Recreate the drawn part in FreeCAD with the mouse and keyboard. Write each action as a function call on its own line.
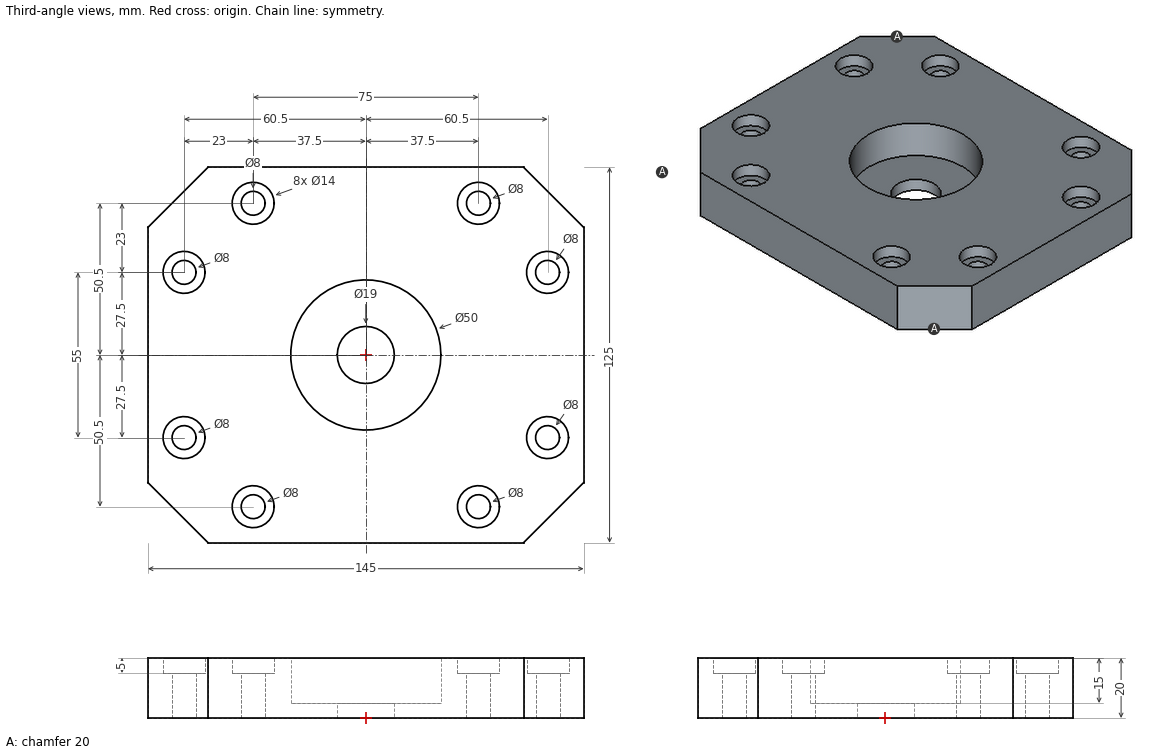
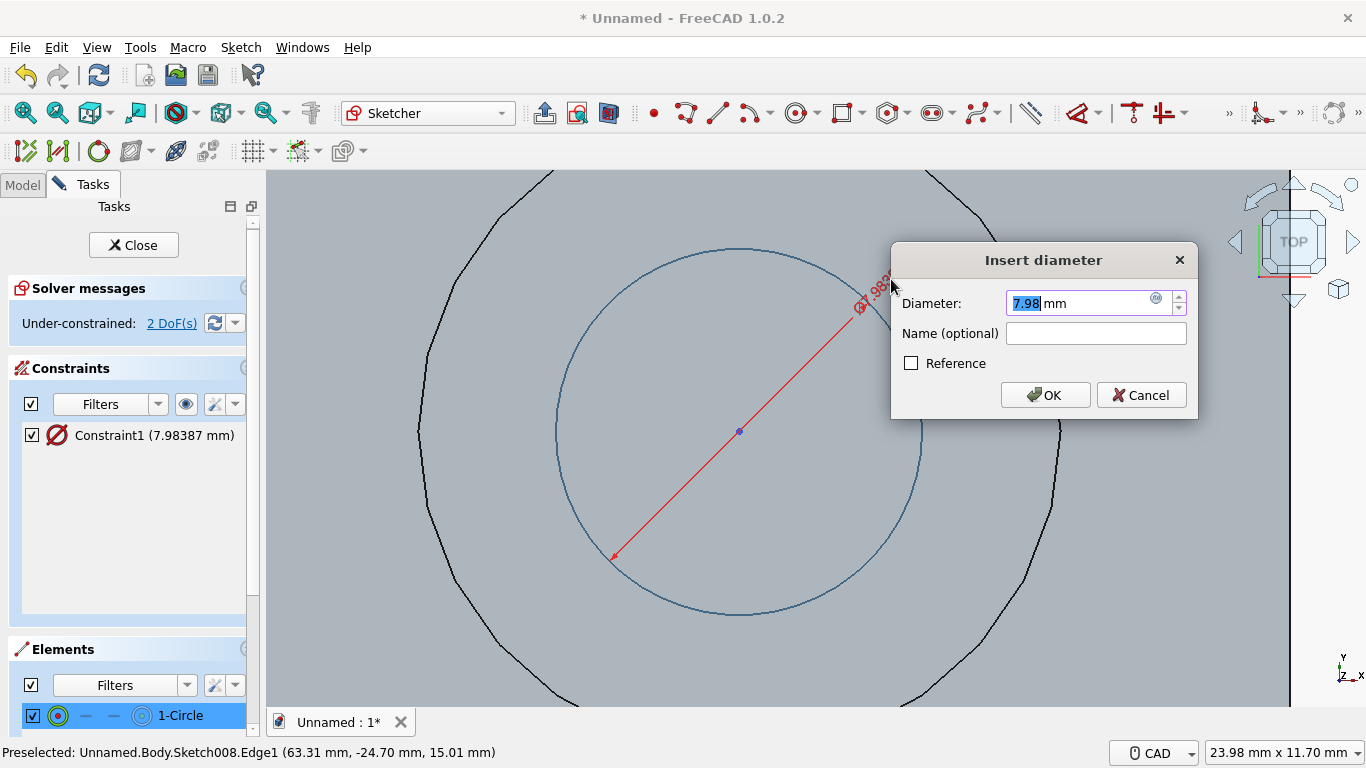
text(8)
key(Return)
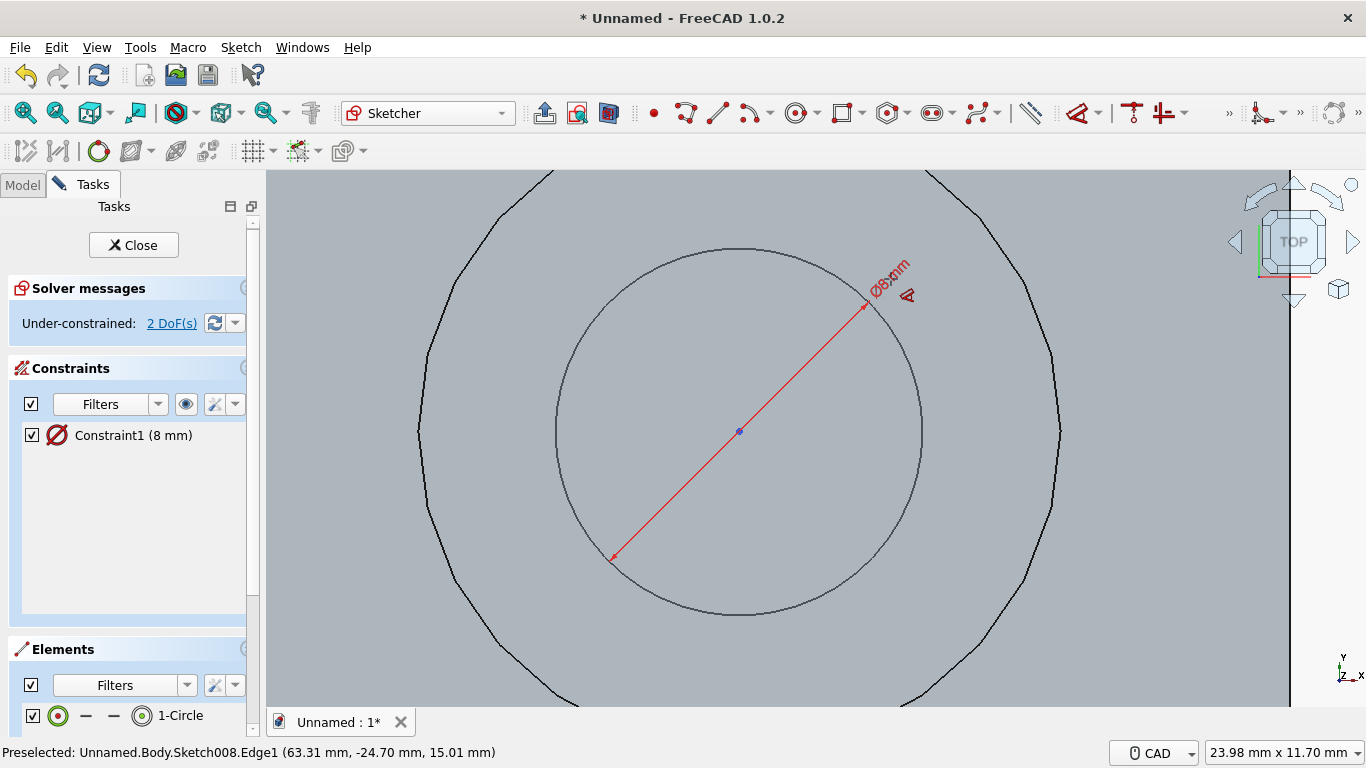
click(739, 432)
click(516, 466)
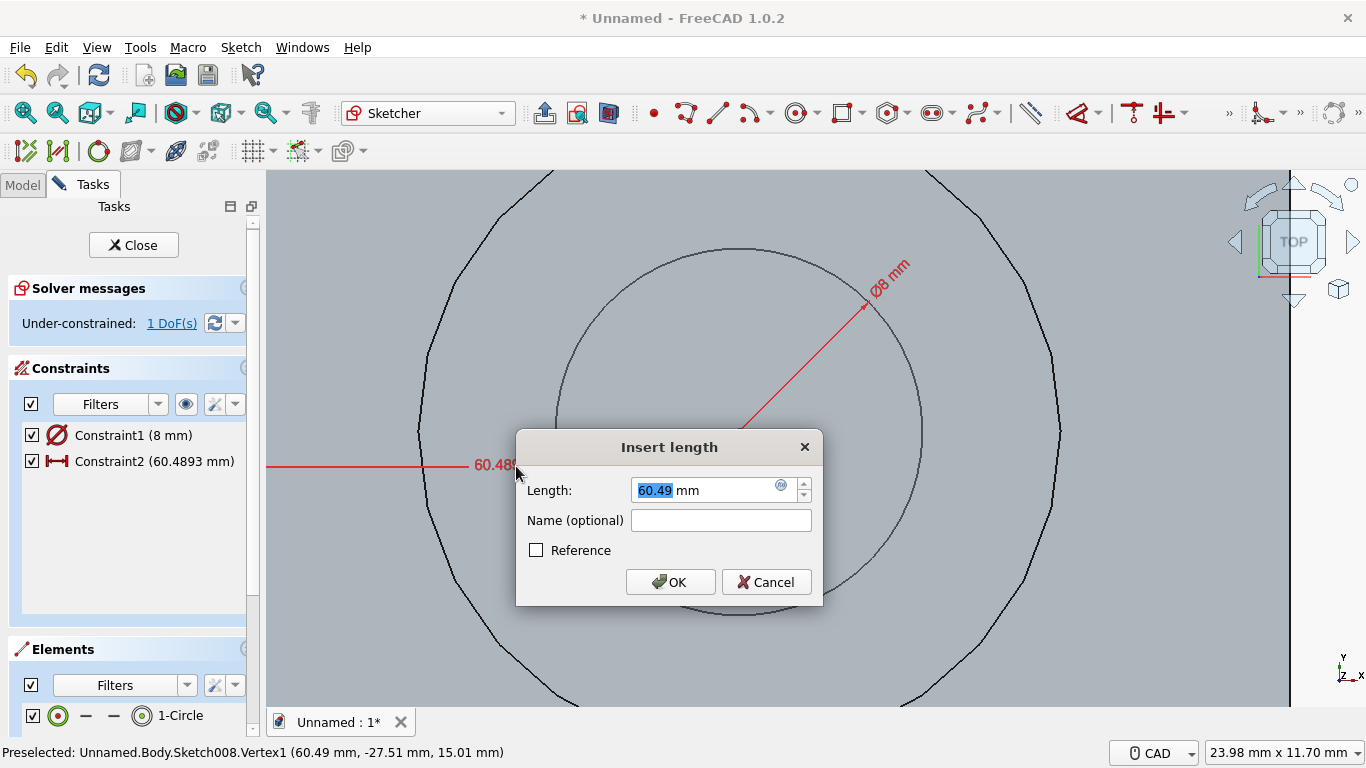
text(60.5)
key(Return)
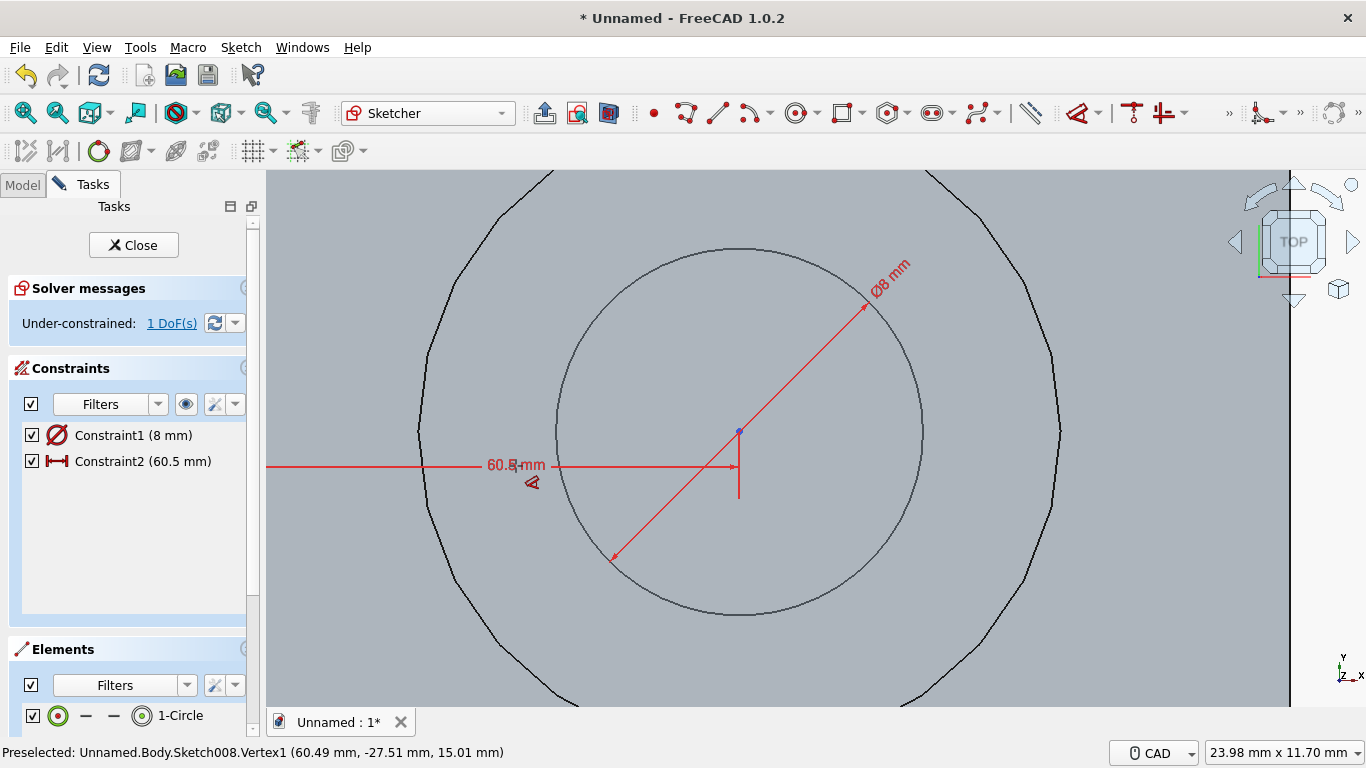
click(739, 432)
click(773, 315)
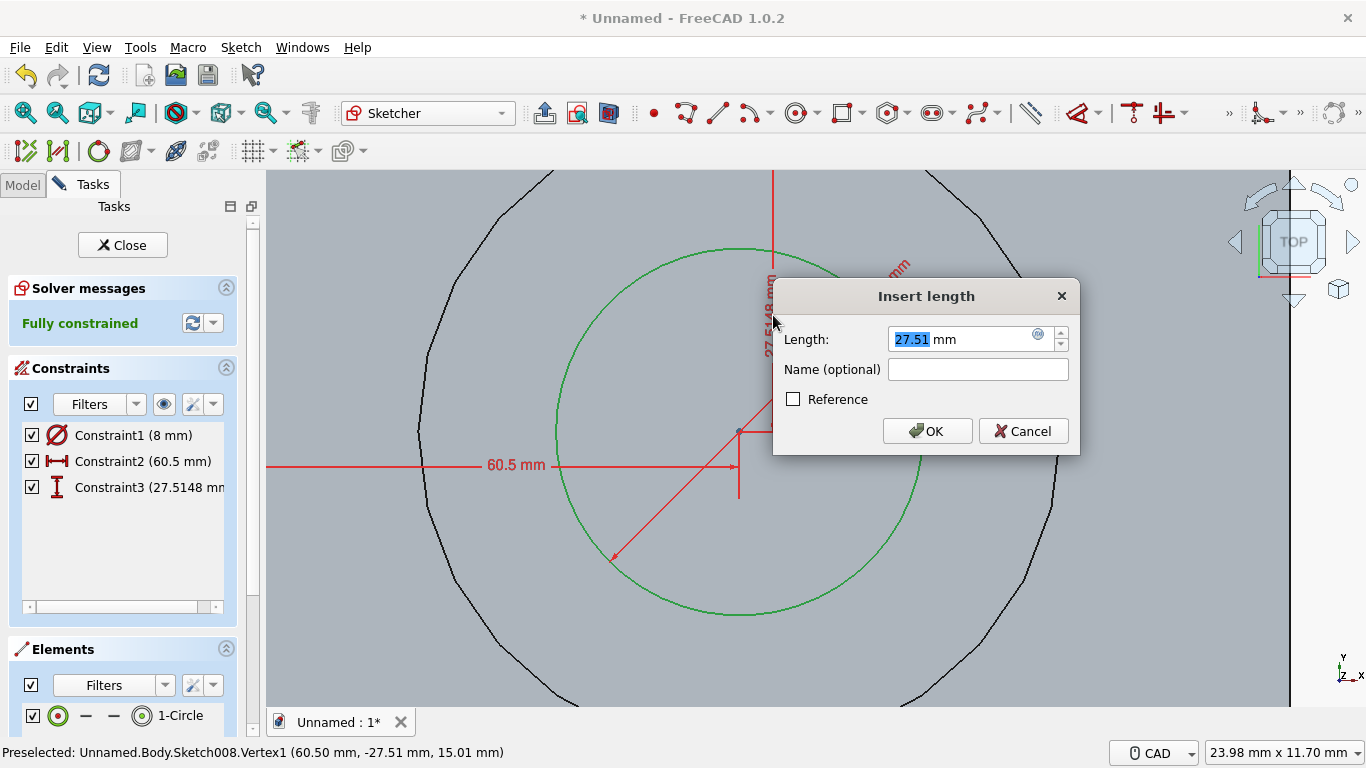
text(27.5)
key(Return)
key(Escape)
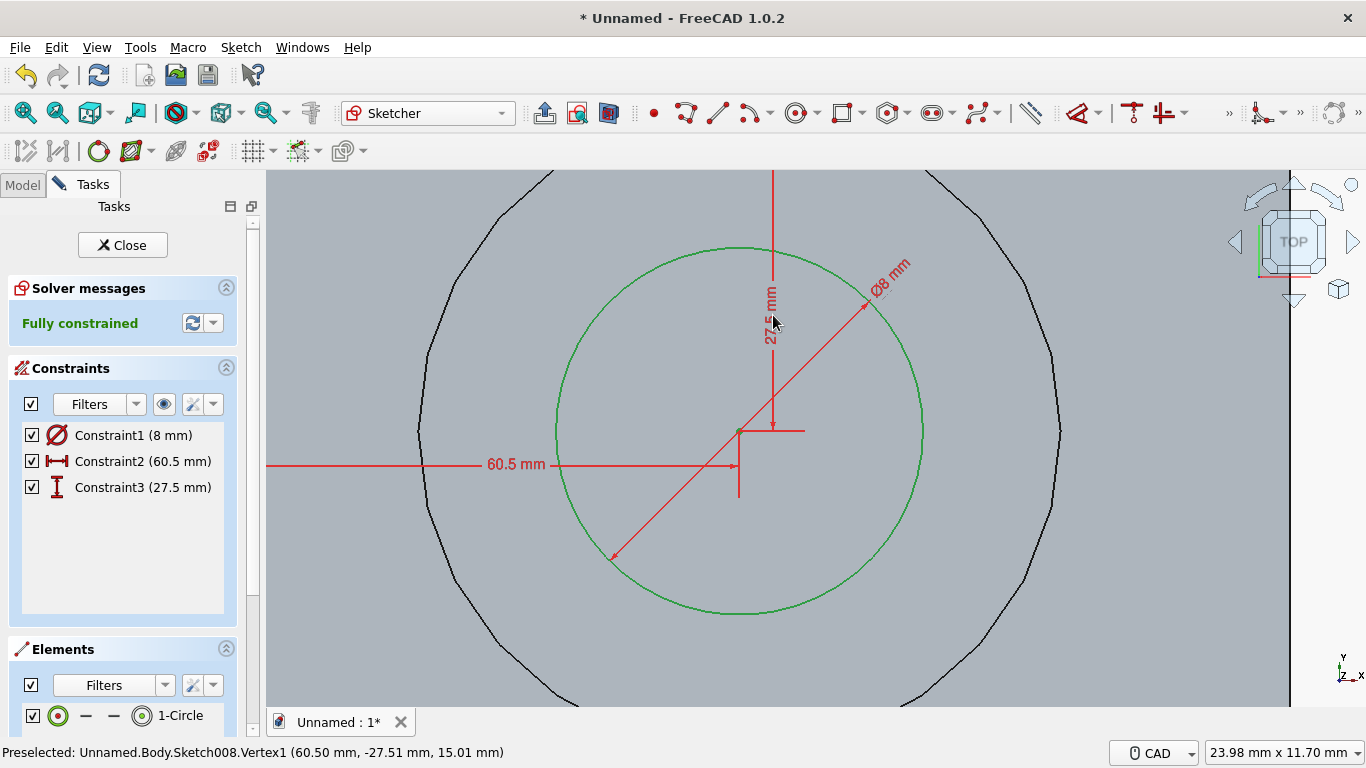
click(123, 245)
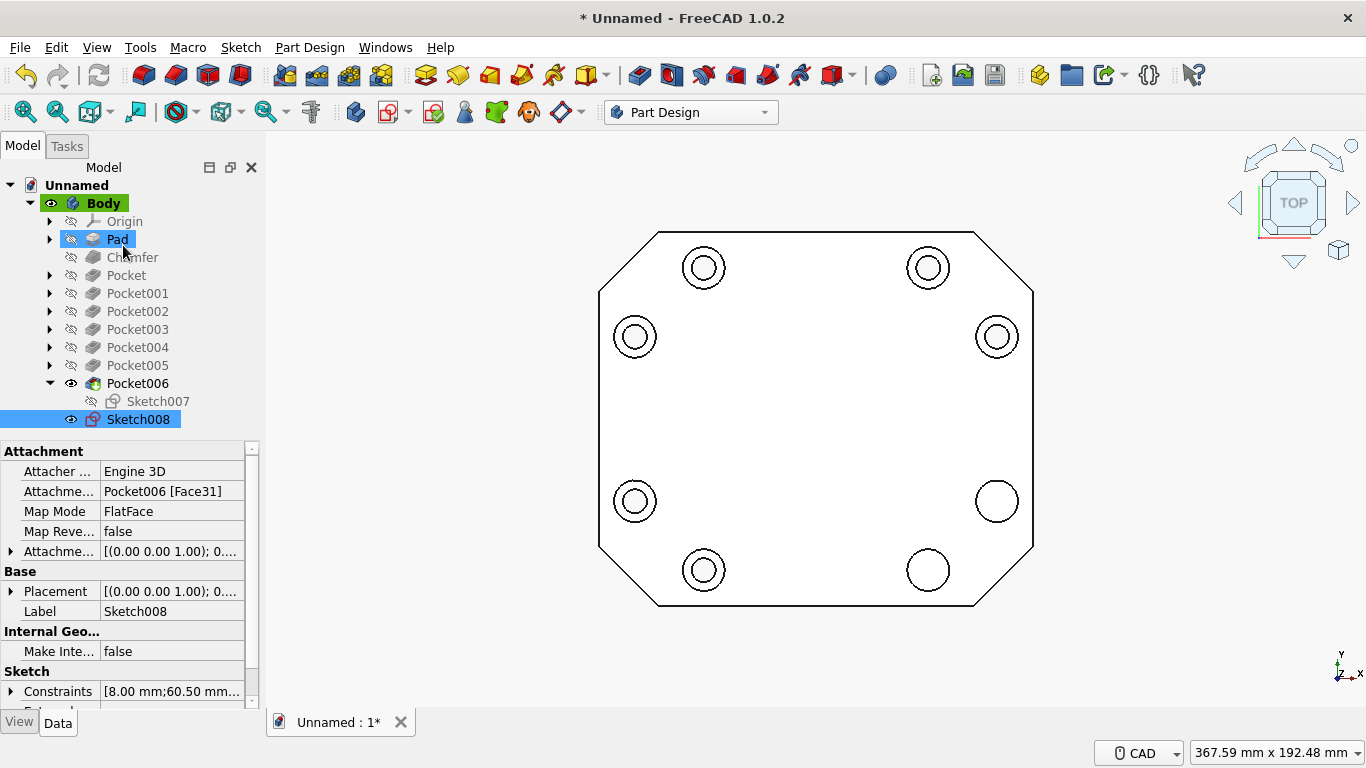
click(640, 76)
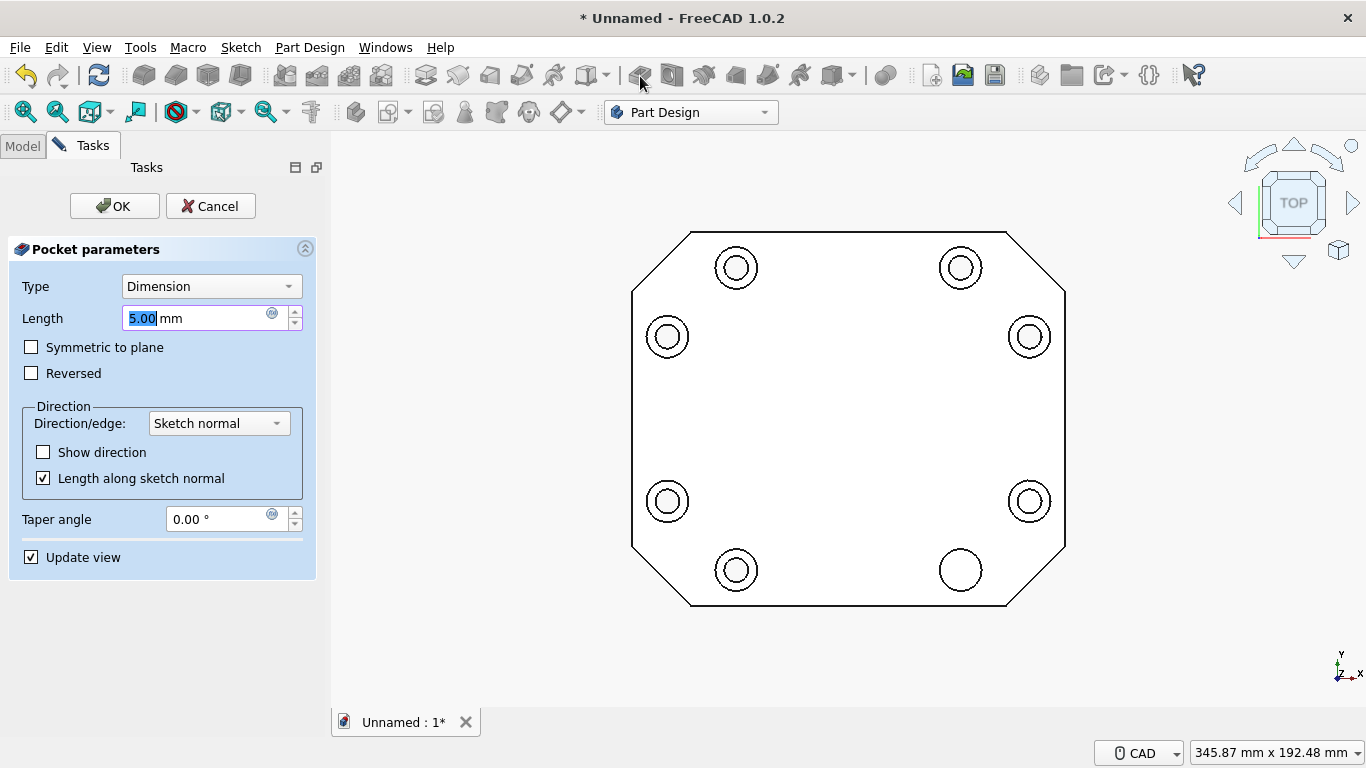
click(212, 286)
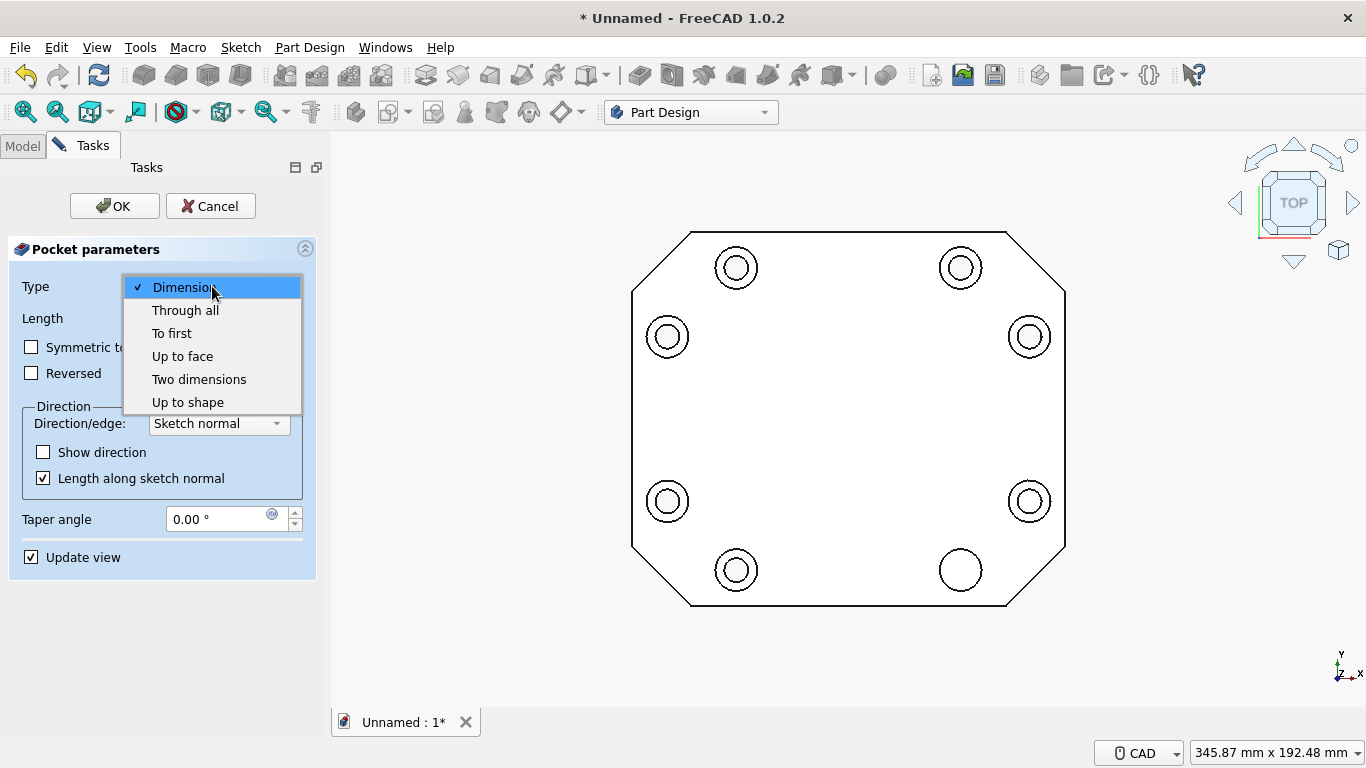
click(212, 334)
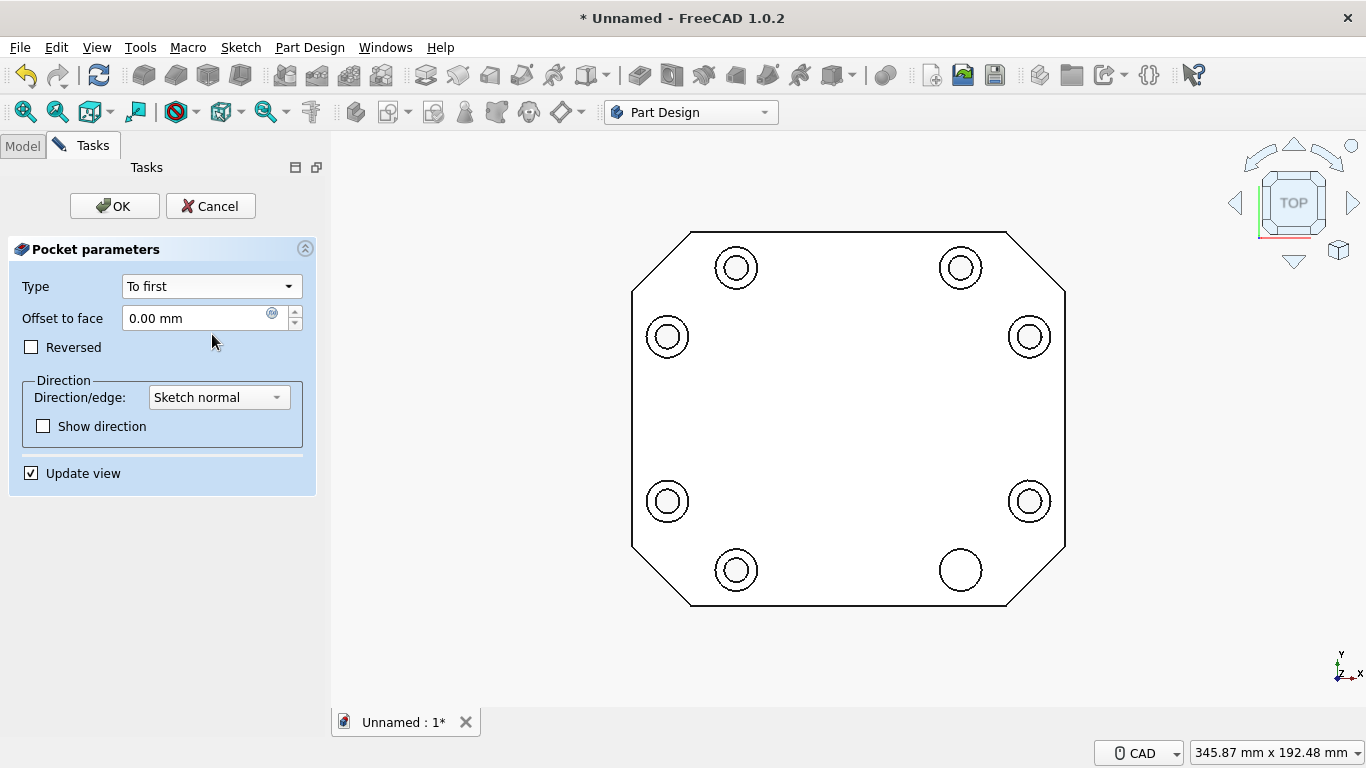
click(115, 206)